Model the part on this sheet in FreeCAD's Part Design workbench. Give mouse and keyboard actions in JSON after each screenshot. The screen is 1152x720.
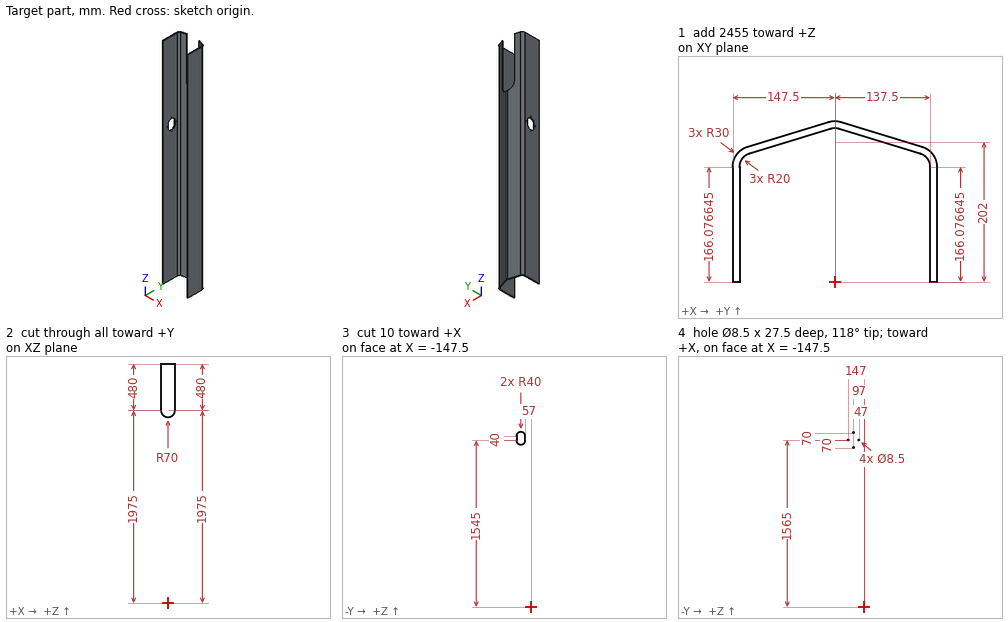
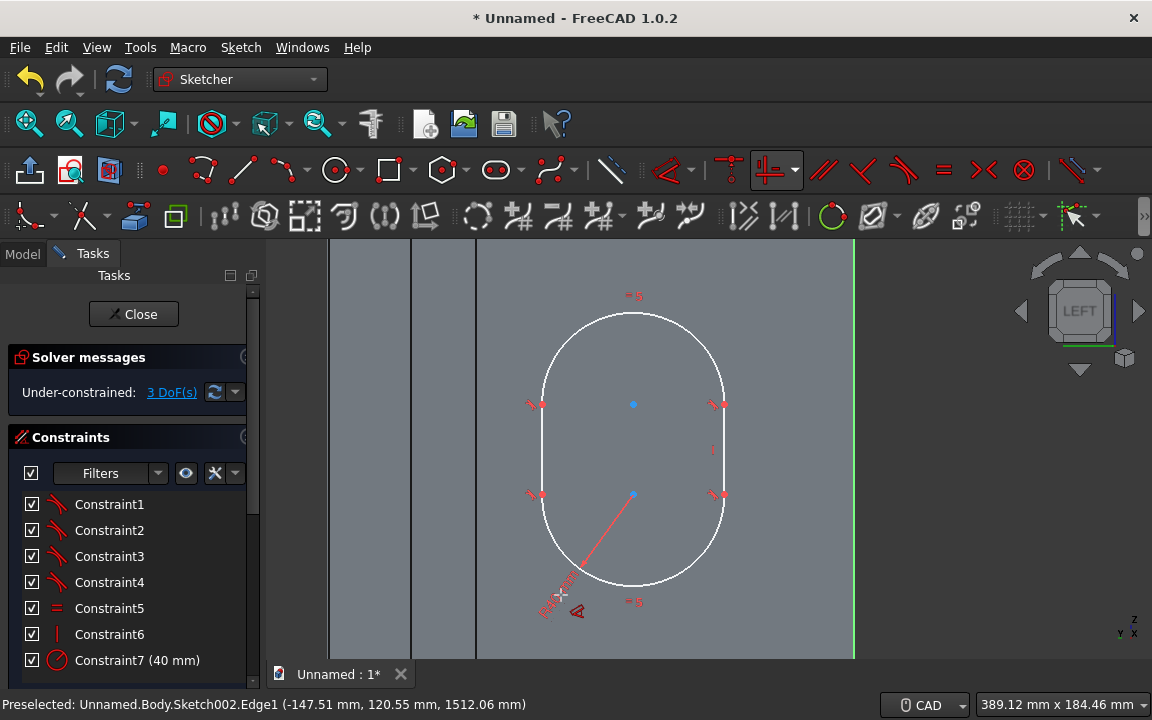
{"action": "left_click", "coordinate": [542, 468]}
{"action": "left_click", "coordinate": [508, 450]}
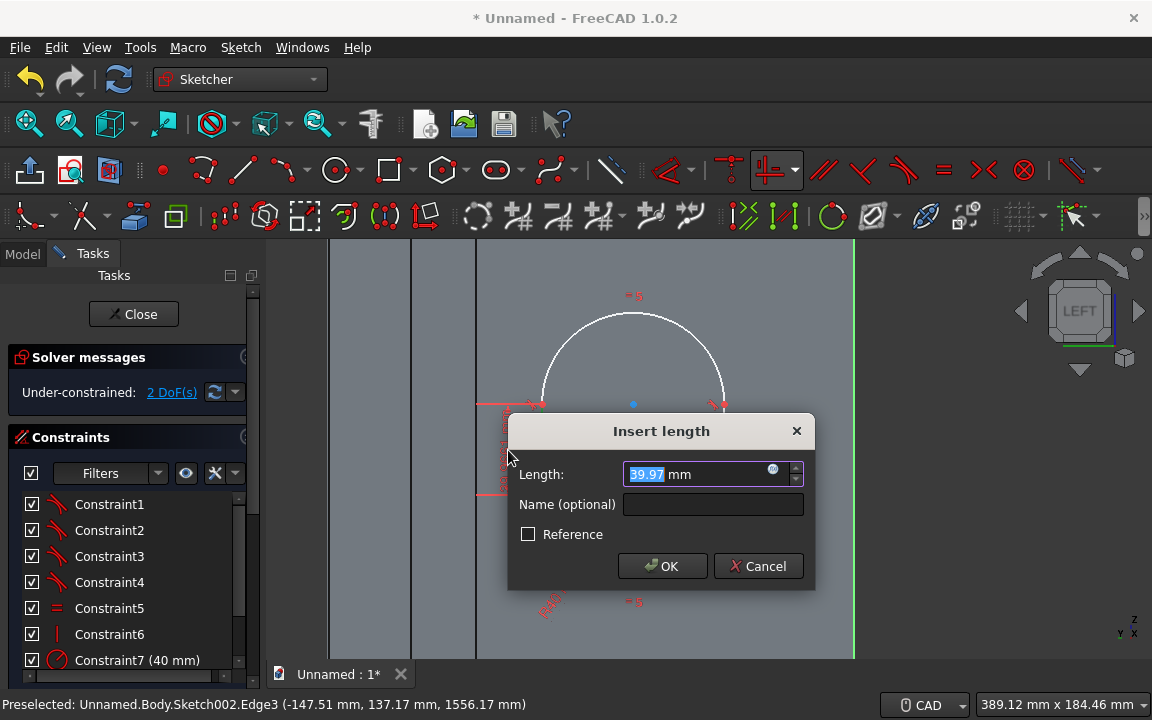
{"action": "type", "text": "40"}
{"action": "key", "text": "Return"}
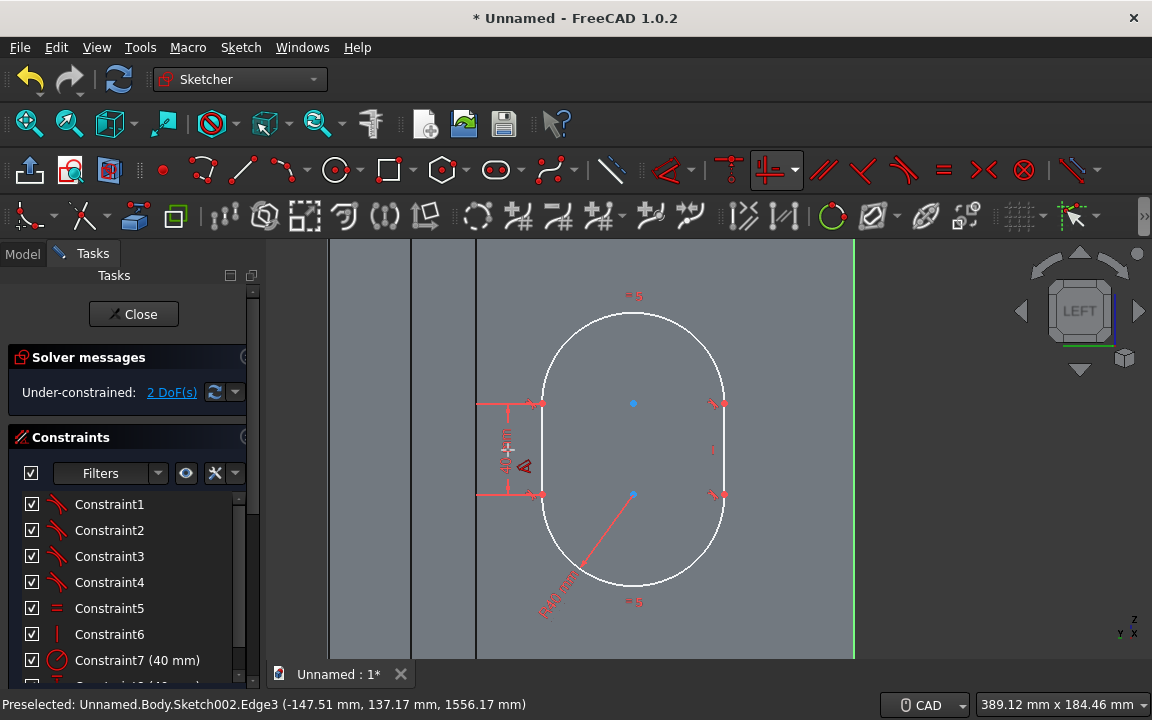
{"action": "left_click", "coordinate": [724, 495]}
{"action": "left_click", "coordinate": [789, 461]}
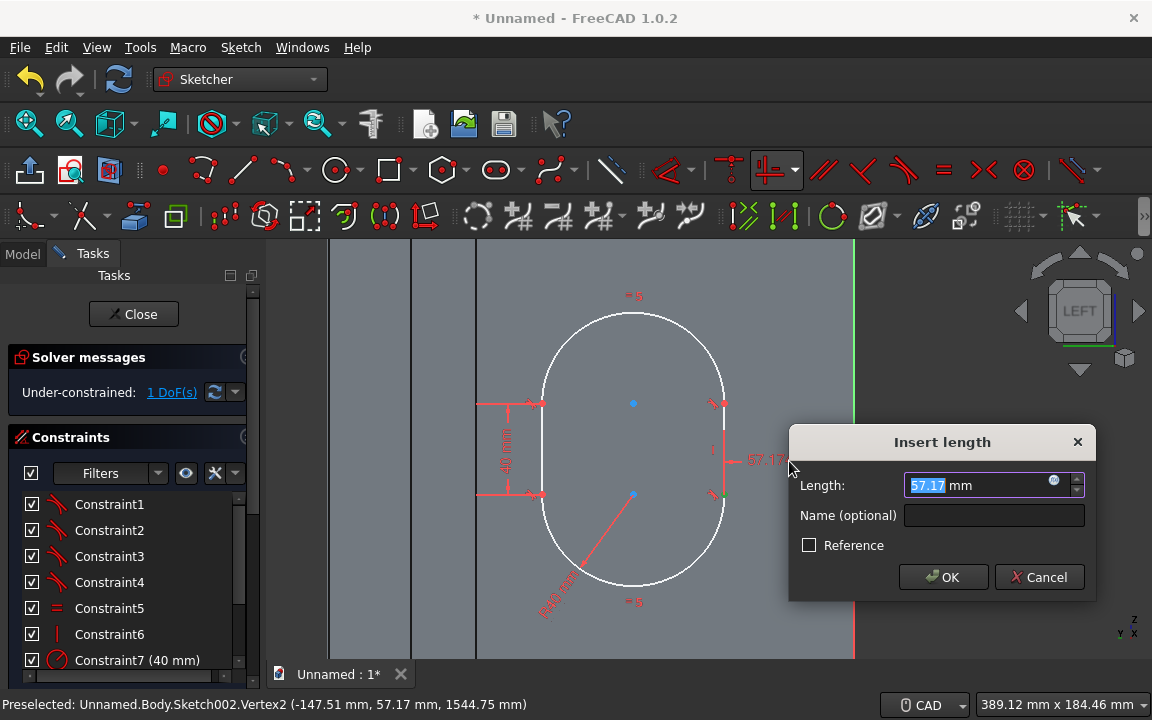
{"action": "type", "text": "57"}
{"action": "key", "text": "Return"}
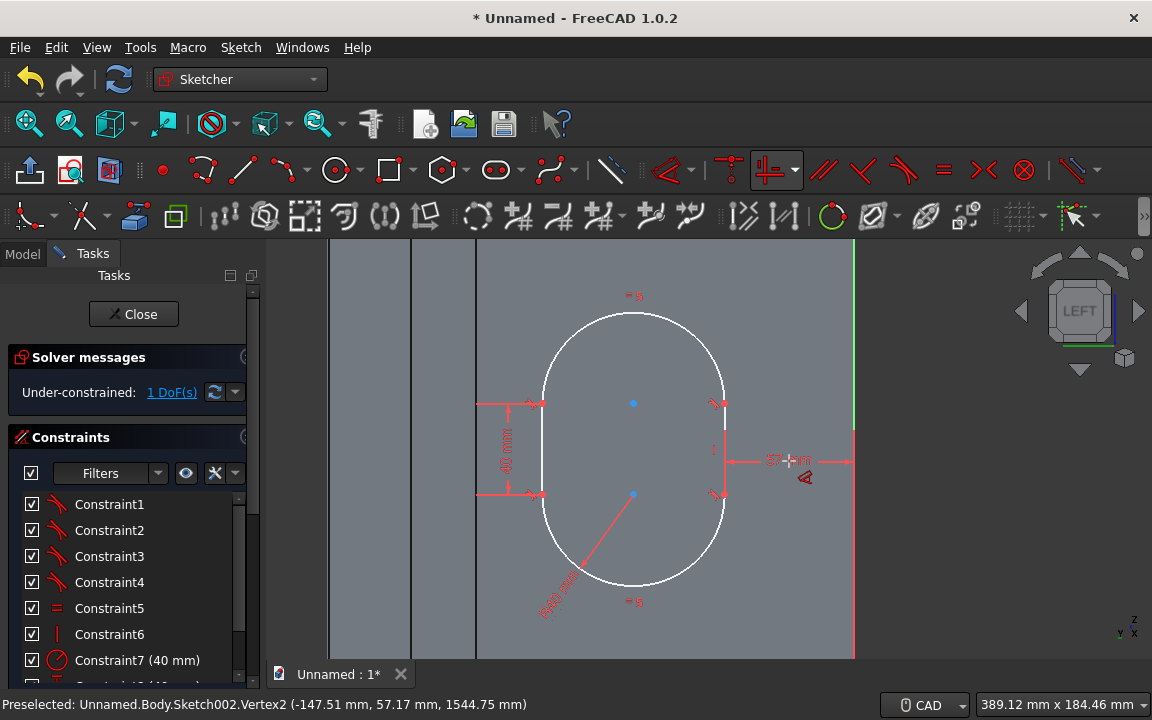
{"action": "left_click", "coordinate": [542, 495]}
{"action": "left_click", "coordinate": [888, 563]}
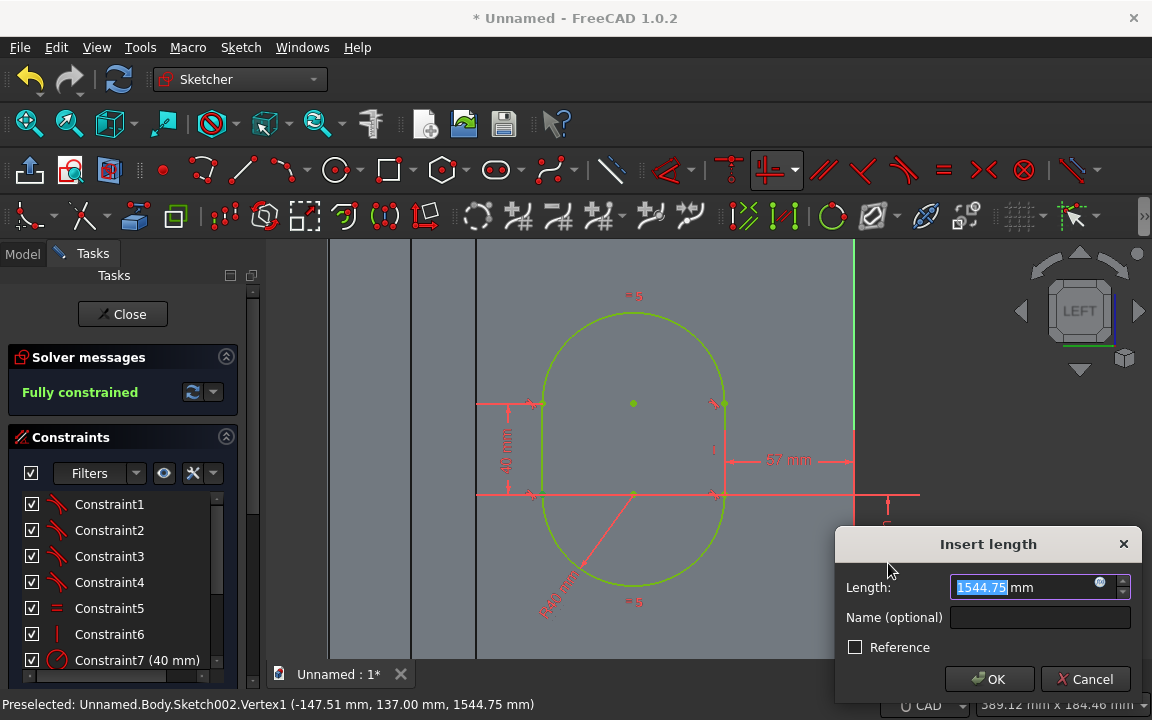
{"action": "type", "text": "1545"}
{"action": "key", "text": "Return"}
{"action": "key", "text": "Escape"}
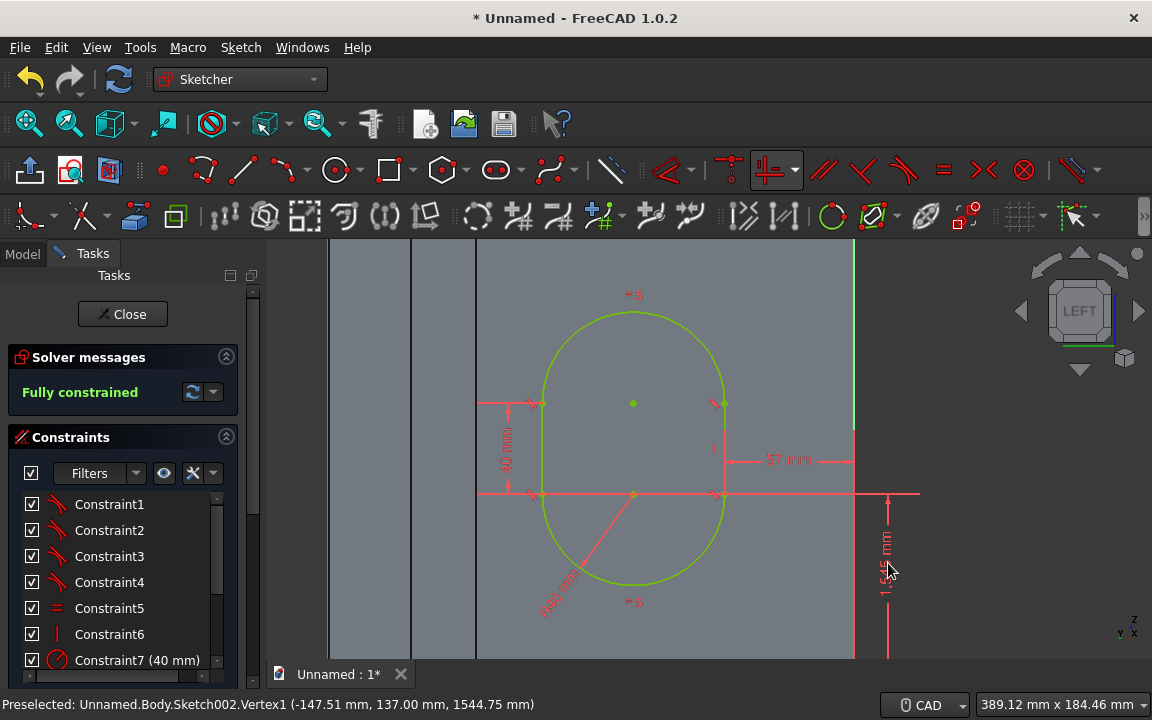
{"action": "left_click", "coordinate": [123, 314]}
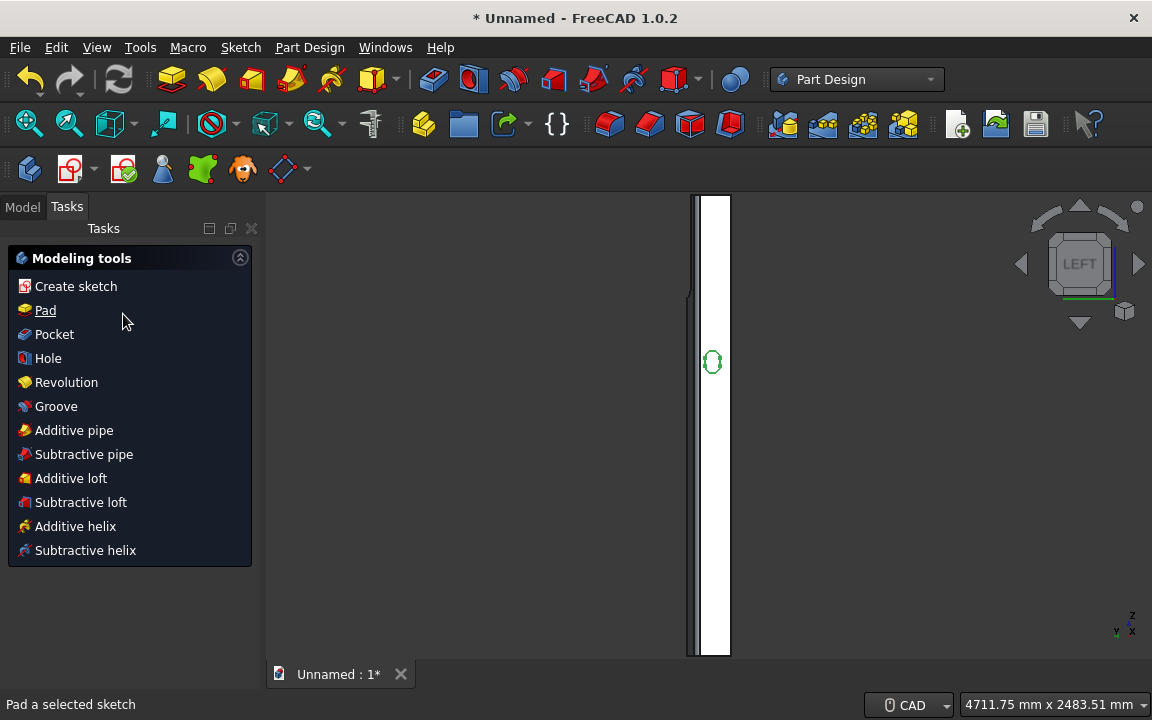
{"action": "left_click", "coordinate": [434, 80]}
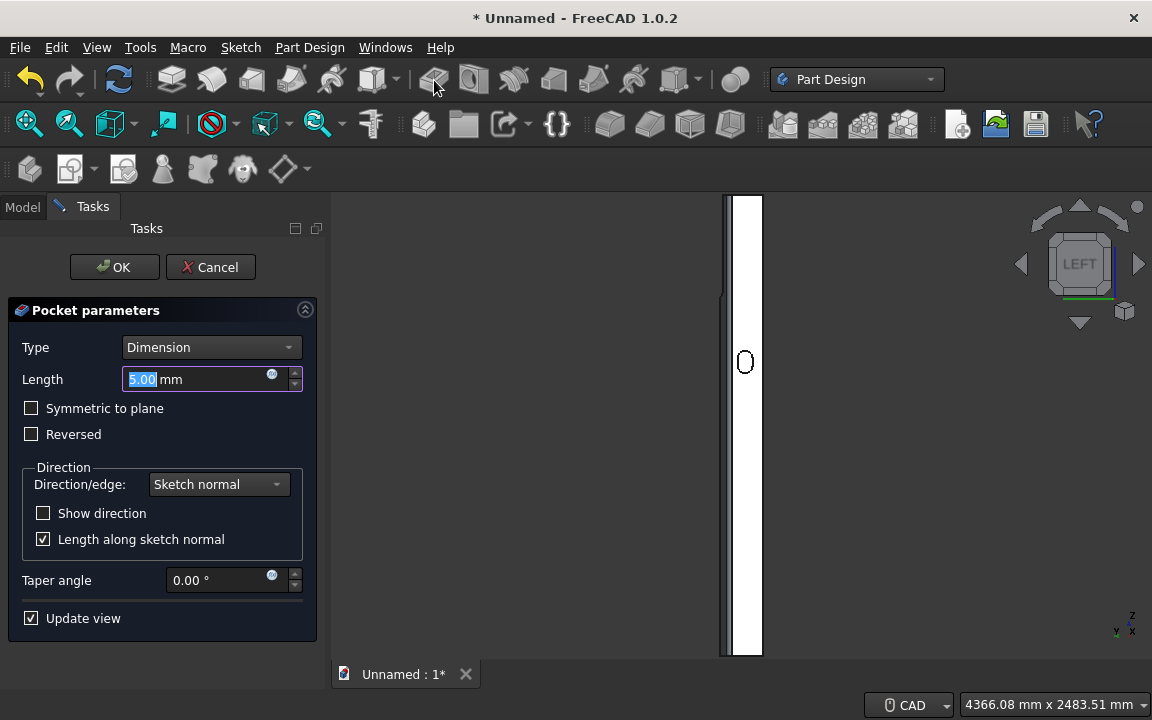
{"action": "type", "text": "10"}
{"action": "key", "text": "Tab"}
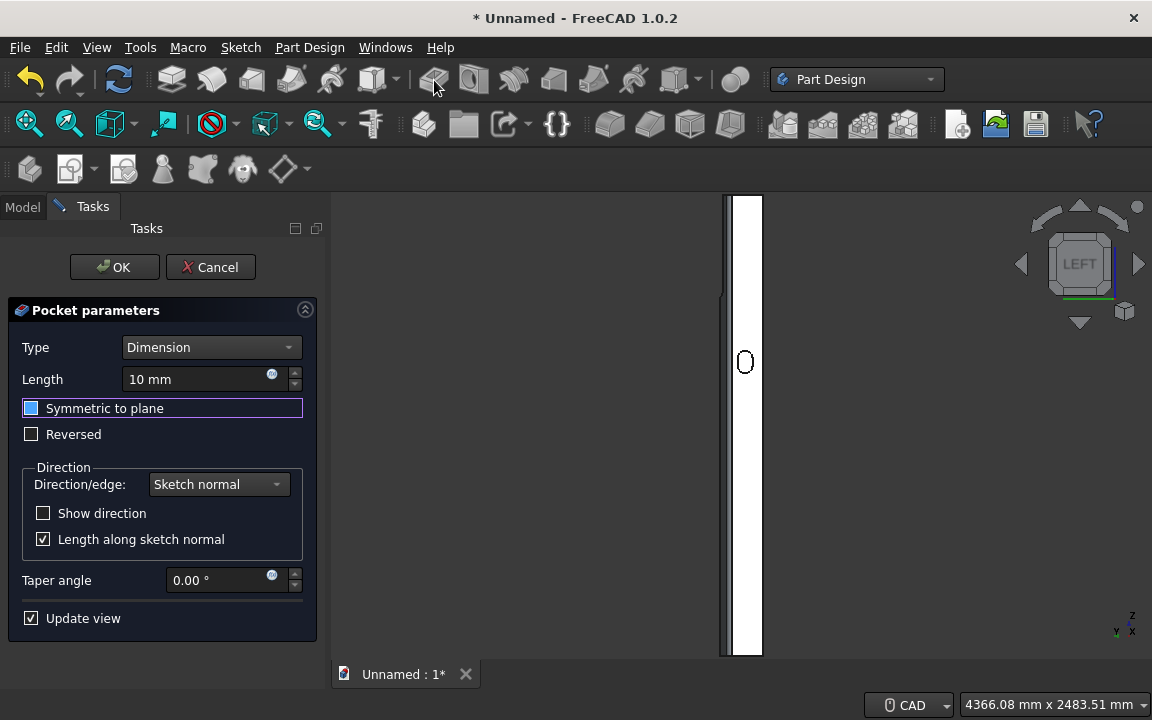
{"action": "left_click", "coordinate": [115, 267]}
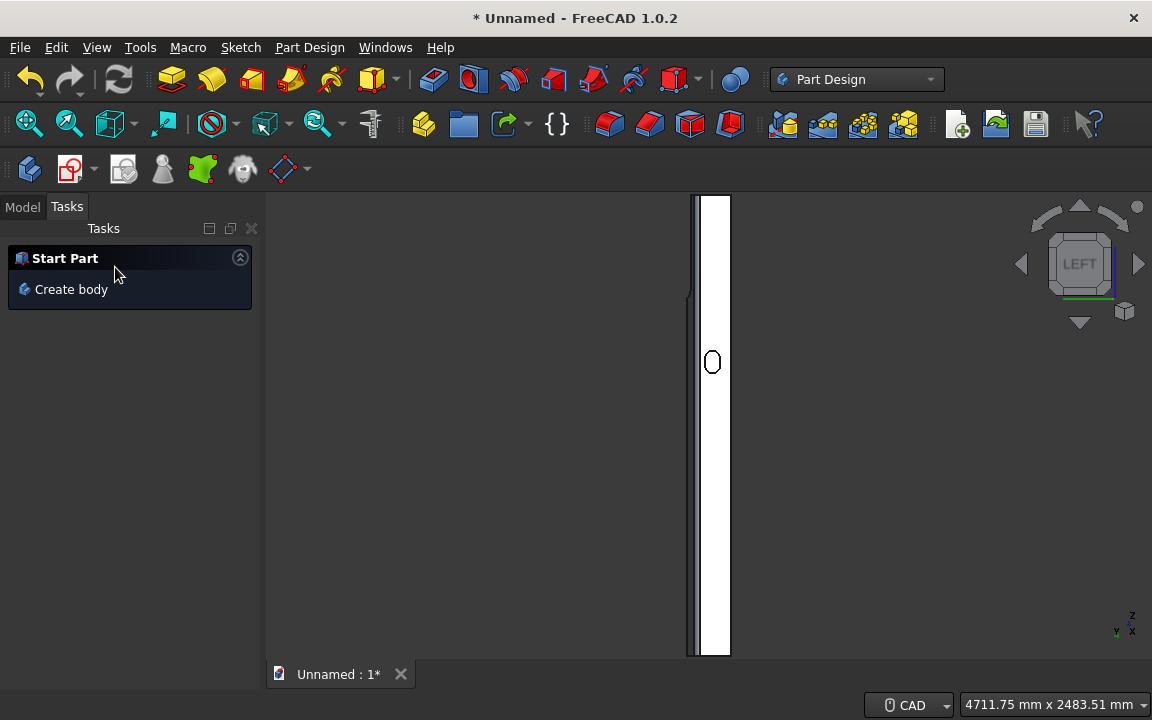
{"action": "left_click", "coordinate": [715, 227]}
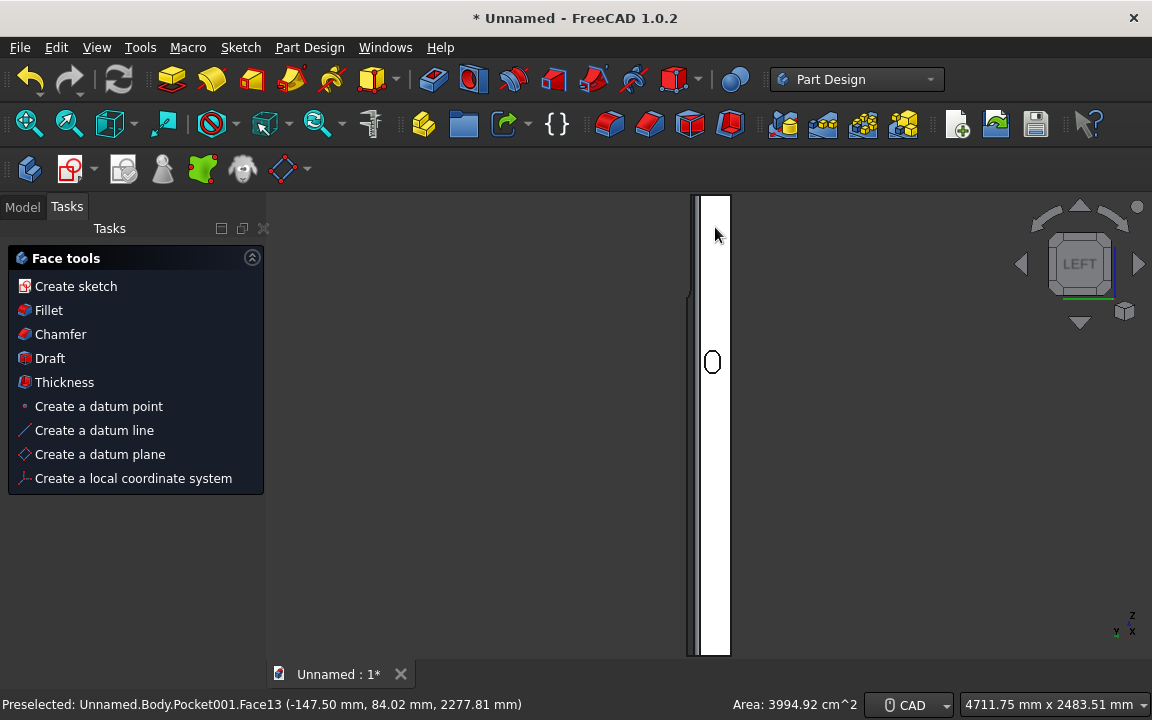
{"action": "left_click", "coordinate": [70, 170]}